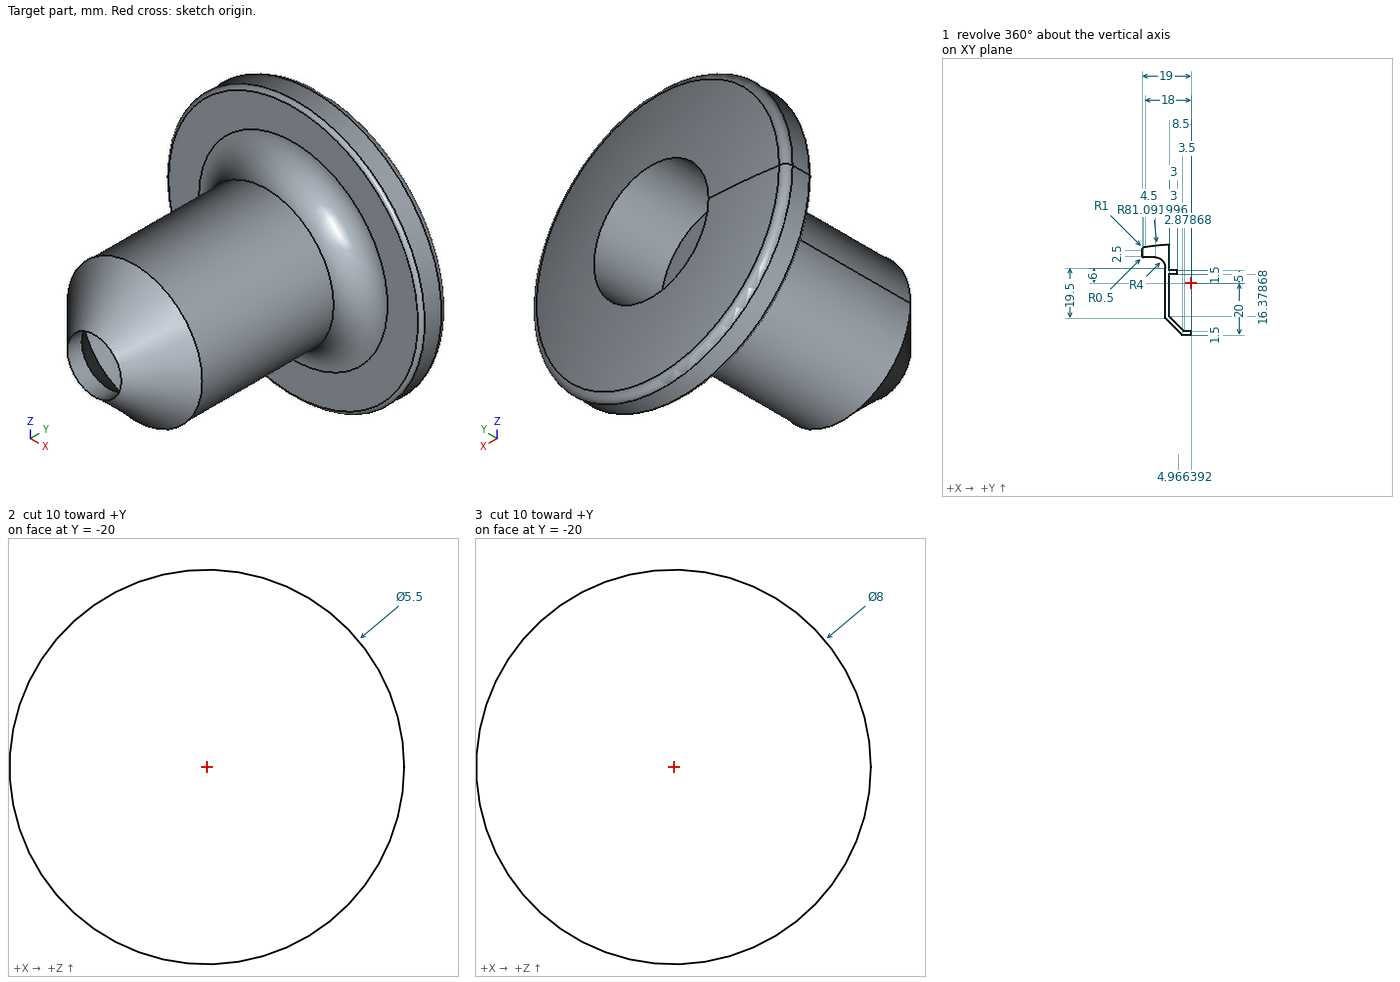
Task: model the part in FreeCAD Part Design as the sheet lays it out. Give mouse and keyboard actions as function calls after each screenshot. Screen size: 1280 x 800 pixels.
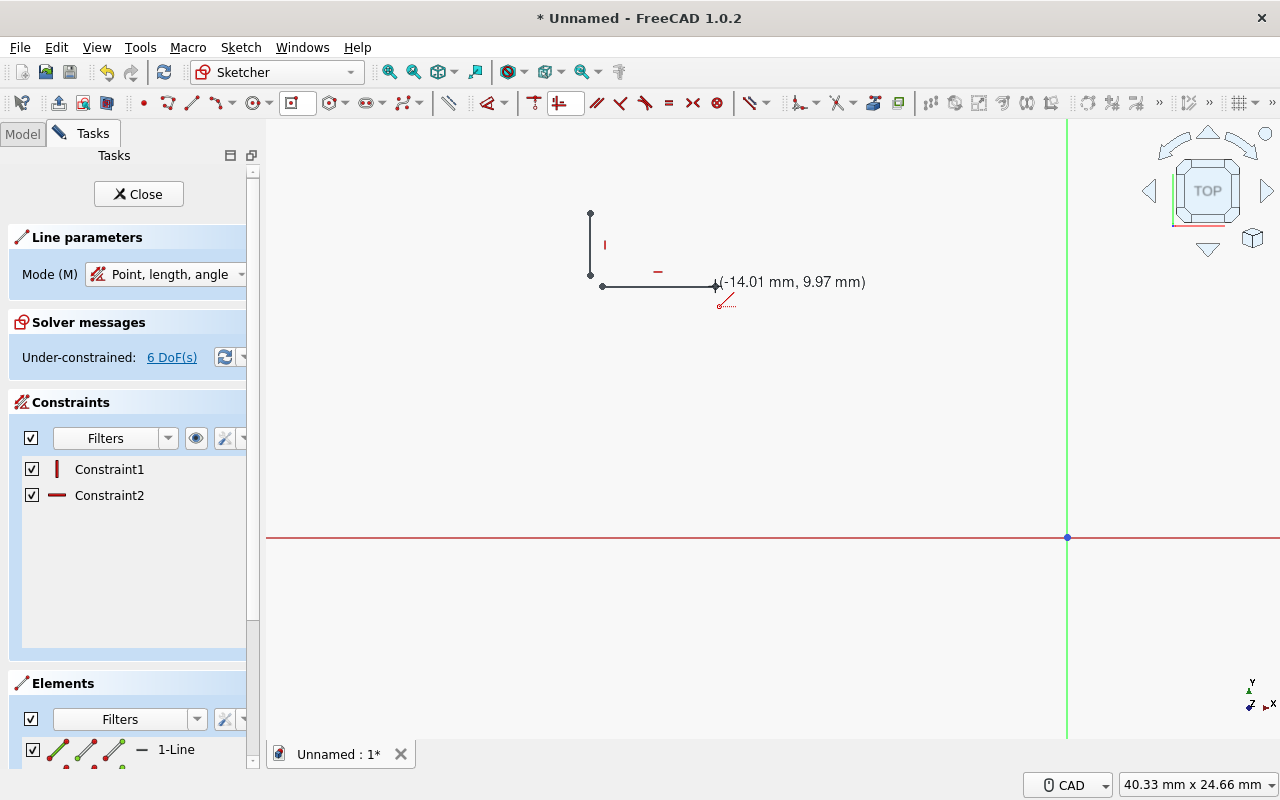
key(g)
key(m)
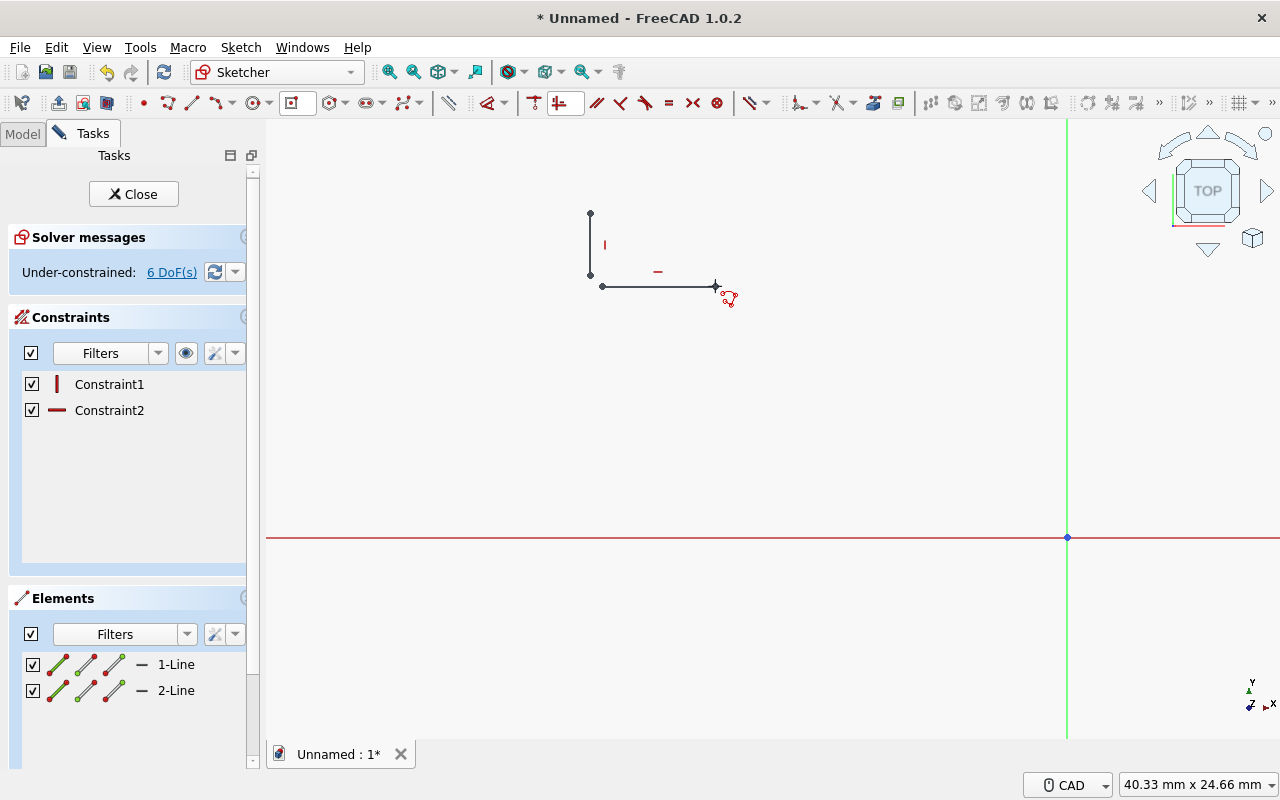
click(816, 387)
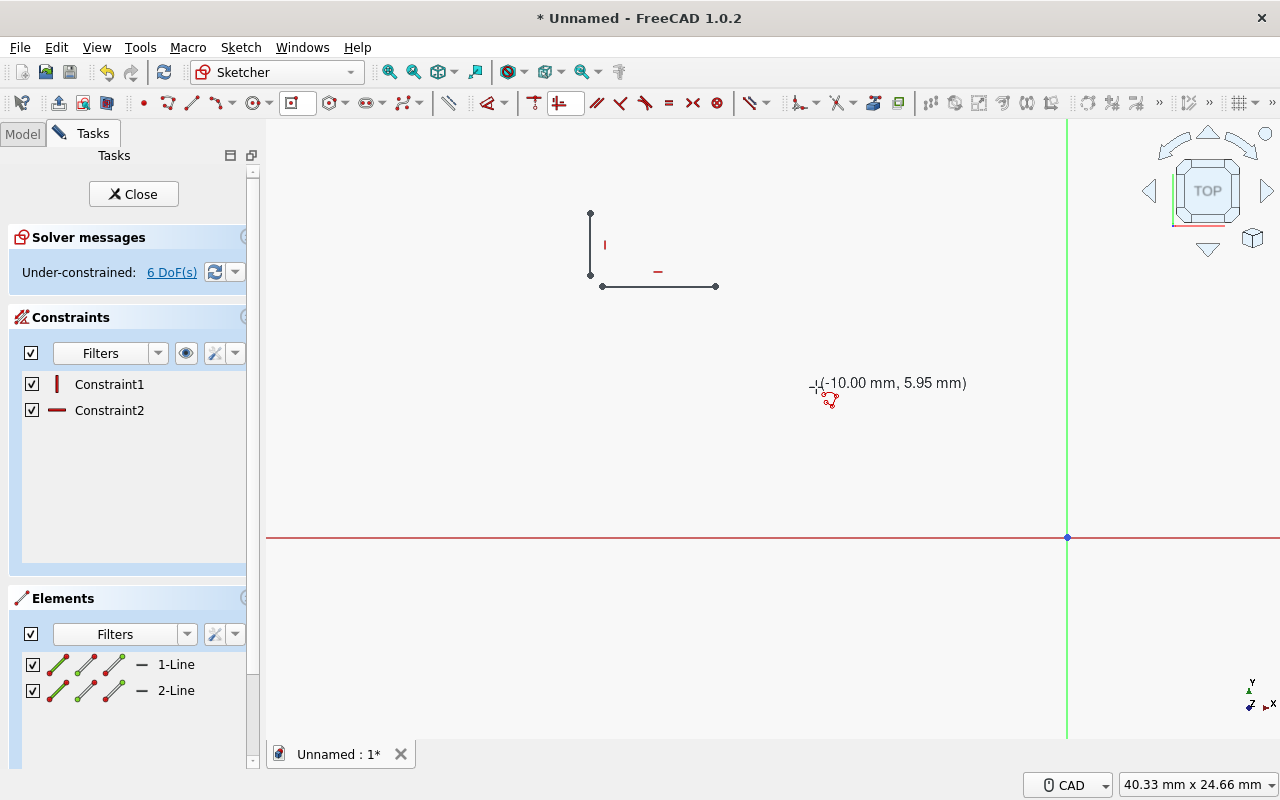
scroll(603, 289, down, 4)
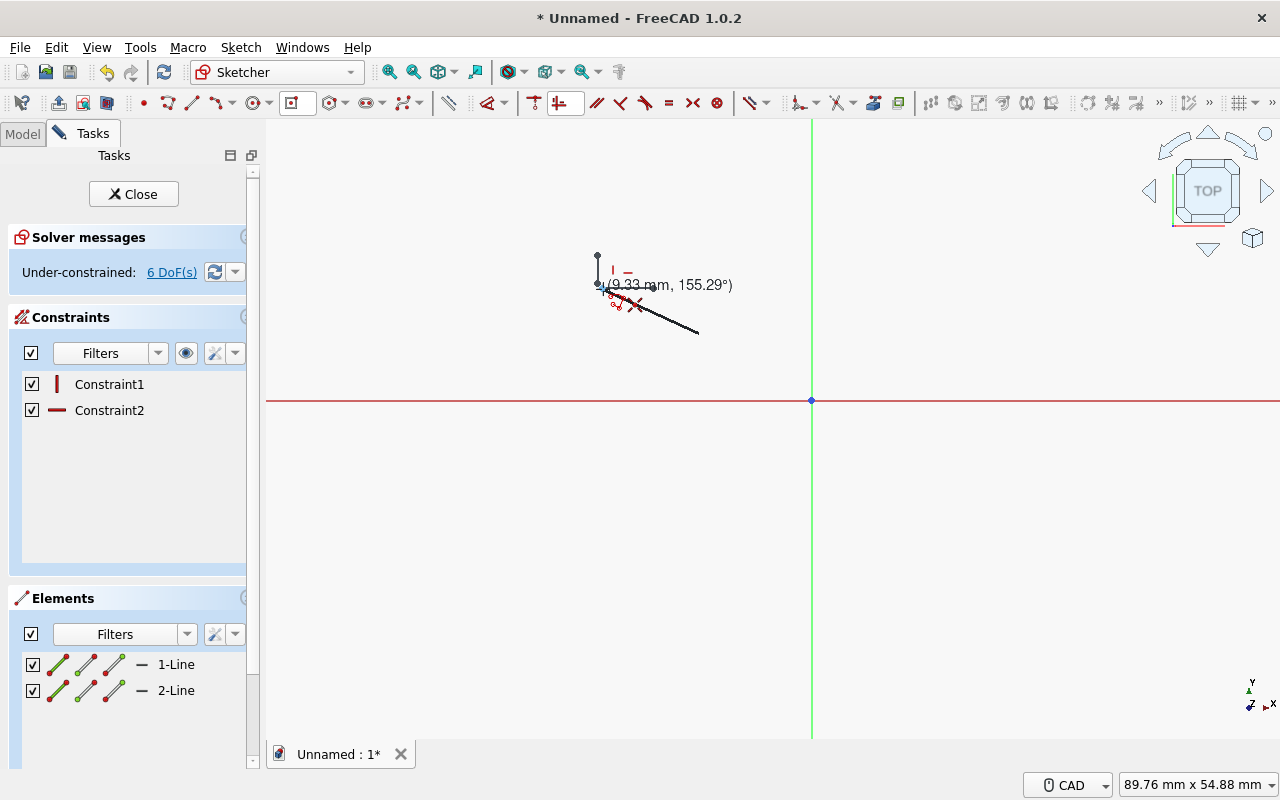
click(699, 553)
click(772, 627)
click(812, 627)
click(803, 610)
click(779, 610)
click(716, 546)
click(716, 361)
click(750, 361)
click(750, 344)
click(716, 344)
click(716, 232)
right_click(716, 232)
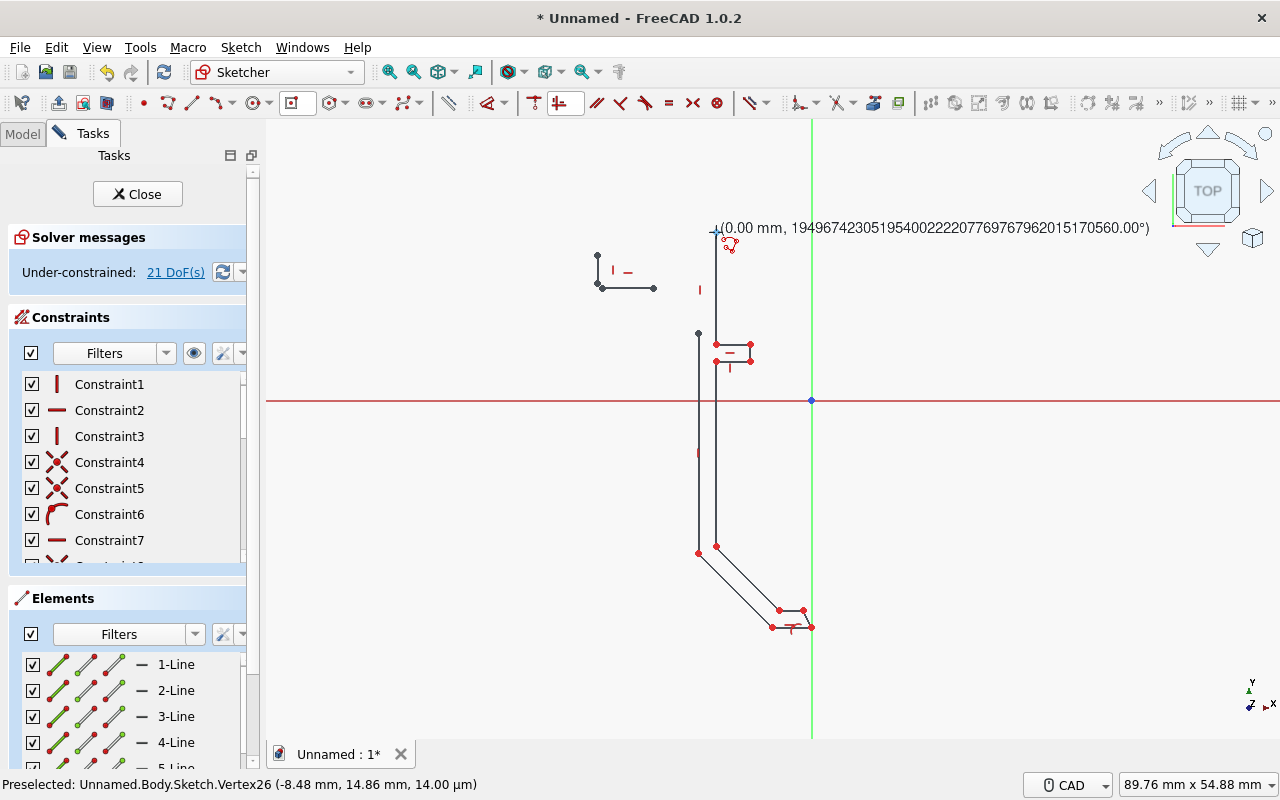
click(216, 104)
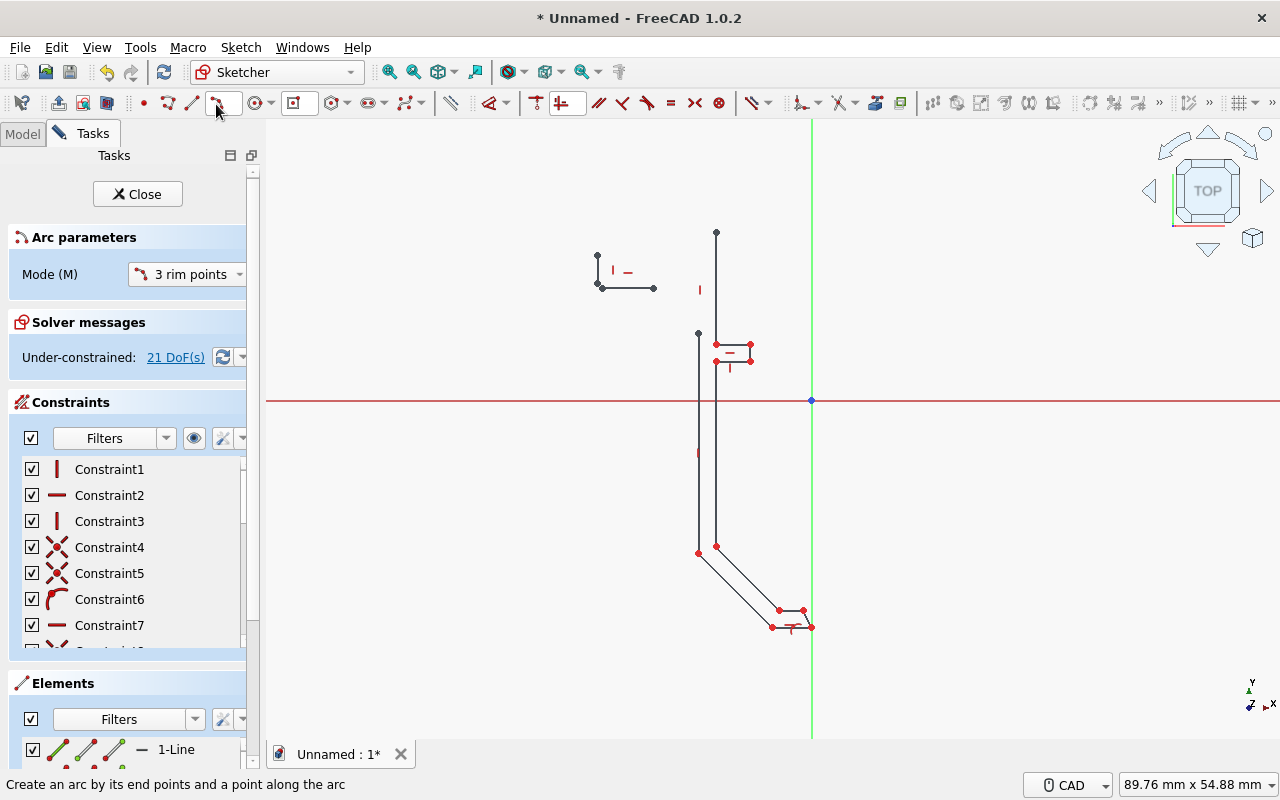
scroll(597, 282, up, 4)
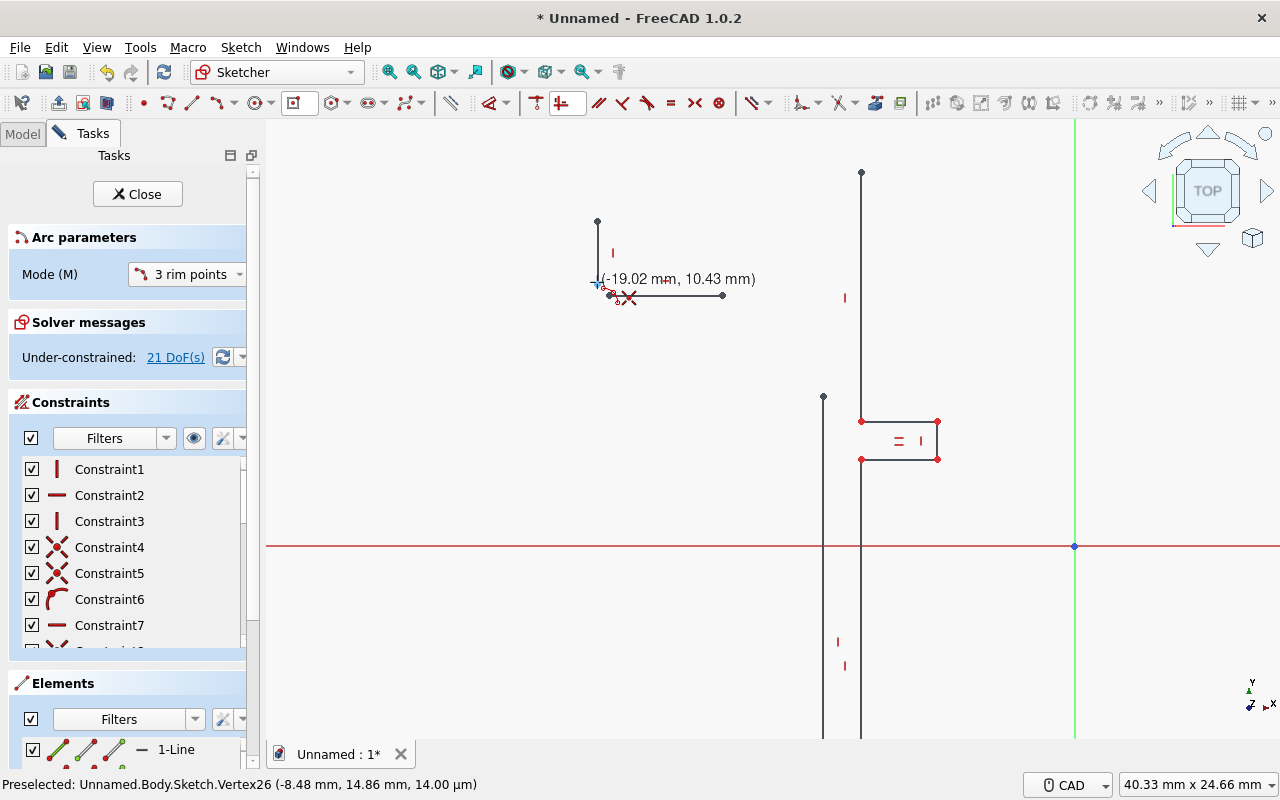
click(598, 284)
click(609, 296)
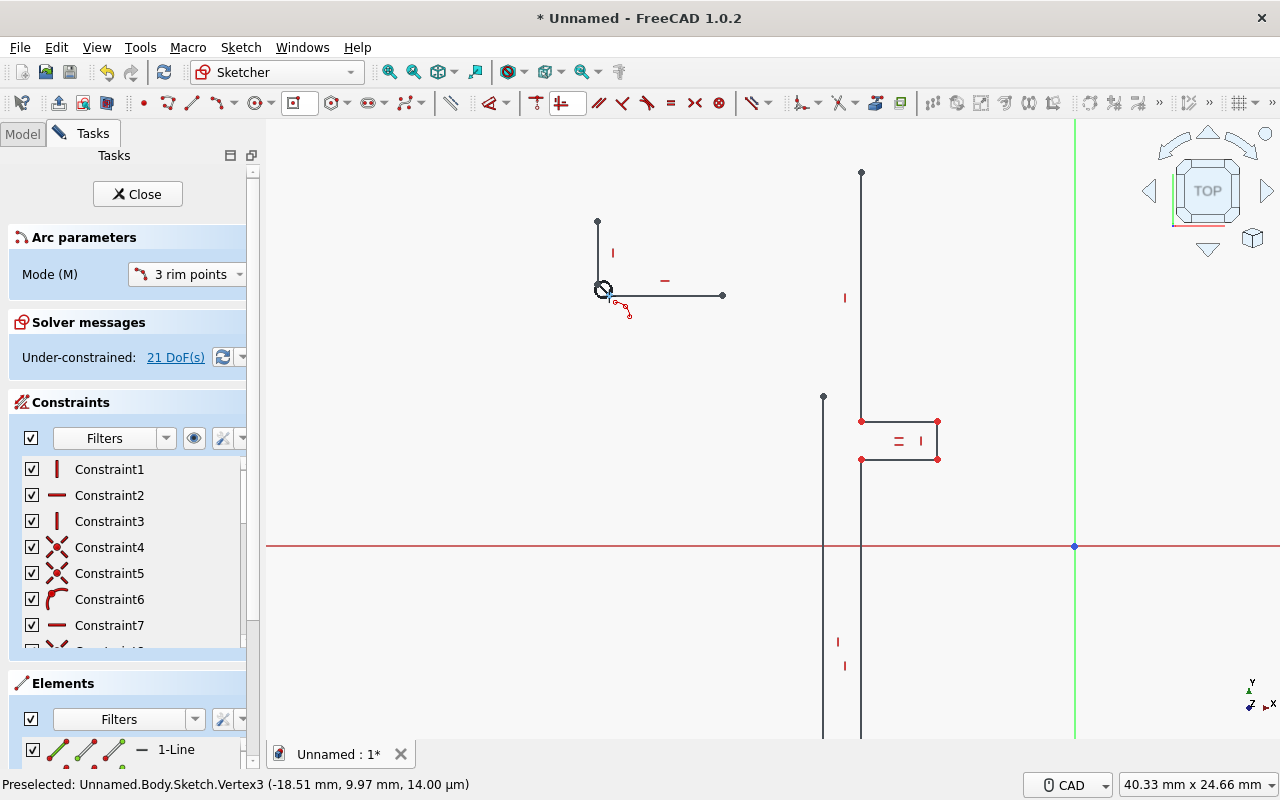
scroll(601, 291, up, 8)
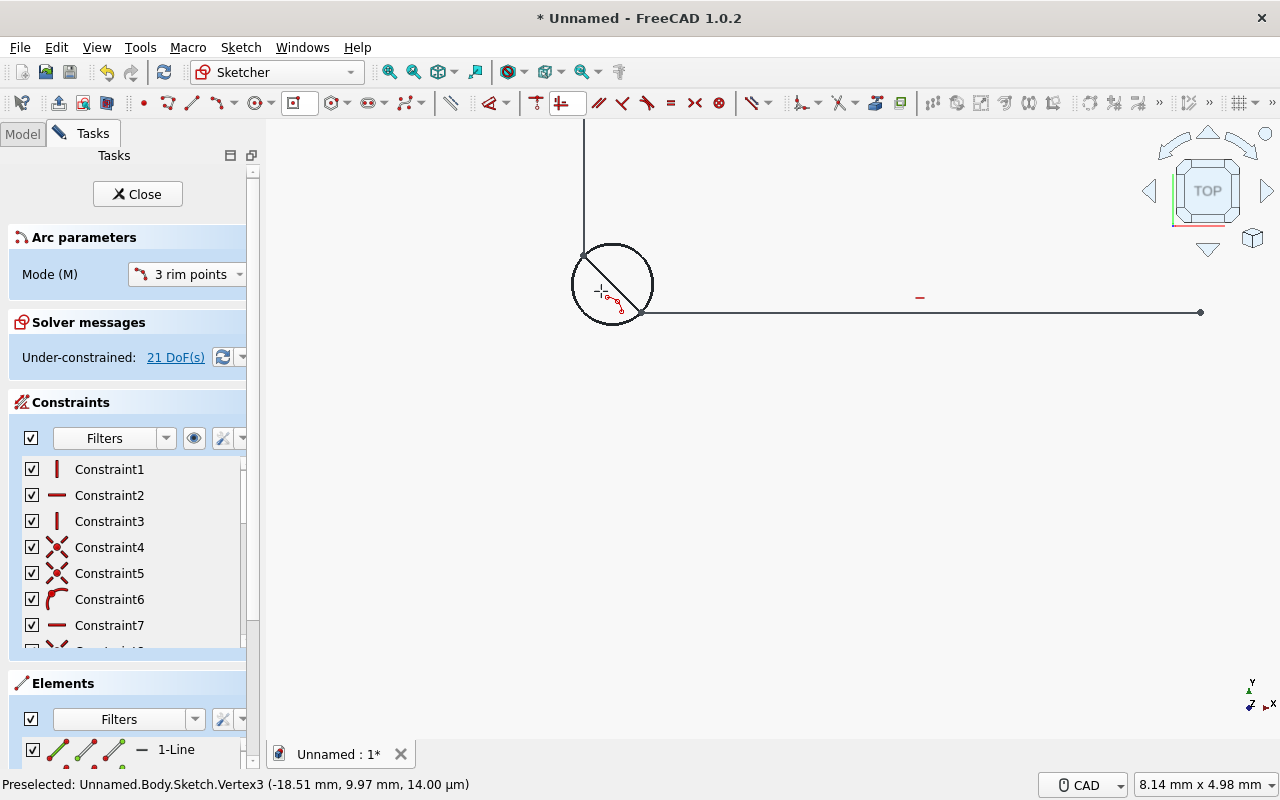
click(598, 291)